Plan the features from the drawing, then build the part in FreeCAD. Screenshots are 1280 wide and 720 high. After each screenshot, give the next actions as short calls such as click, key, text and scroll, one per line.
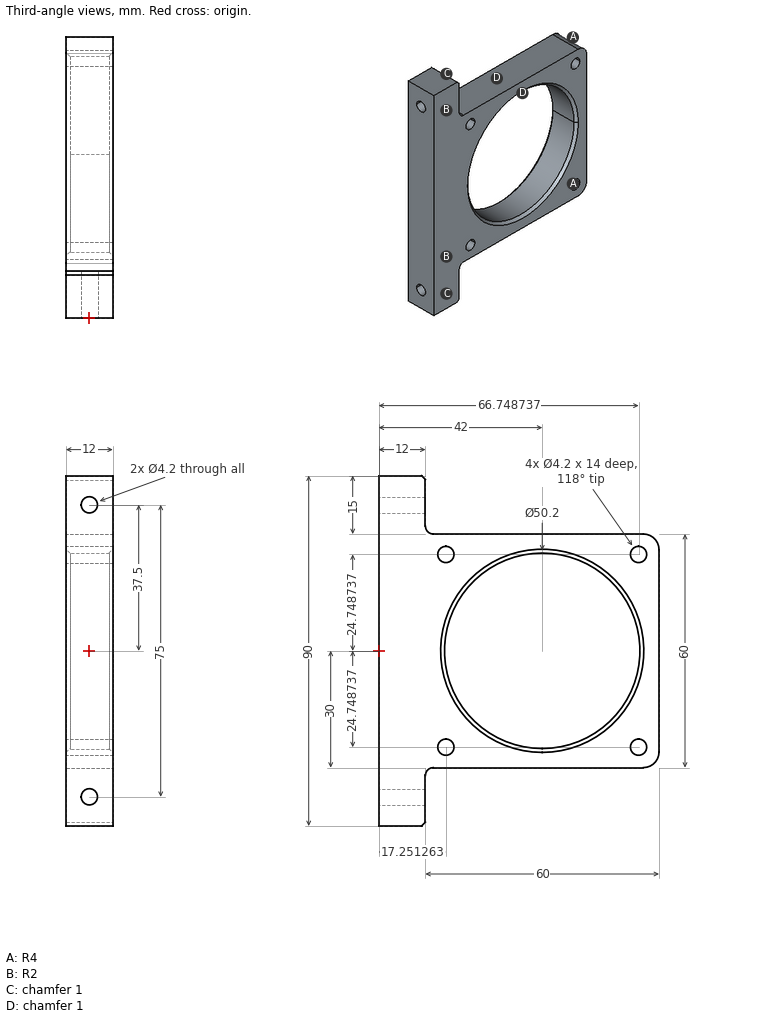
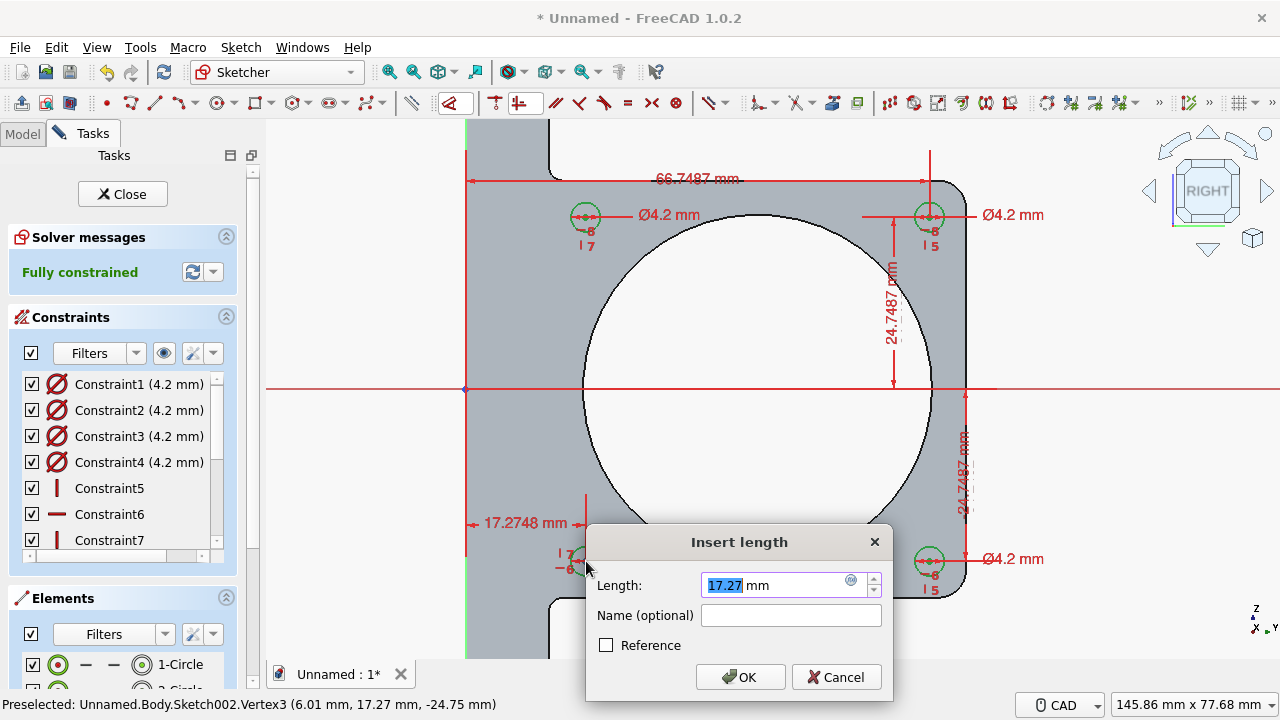
text(17.251263)
key(Return)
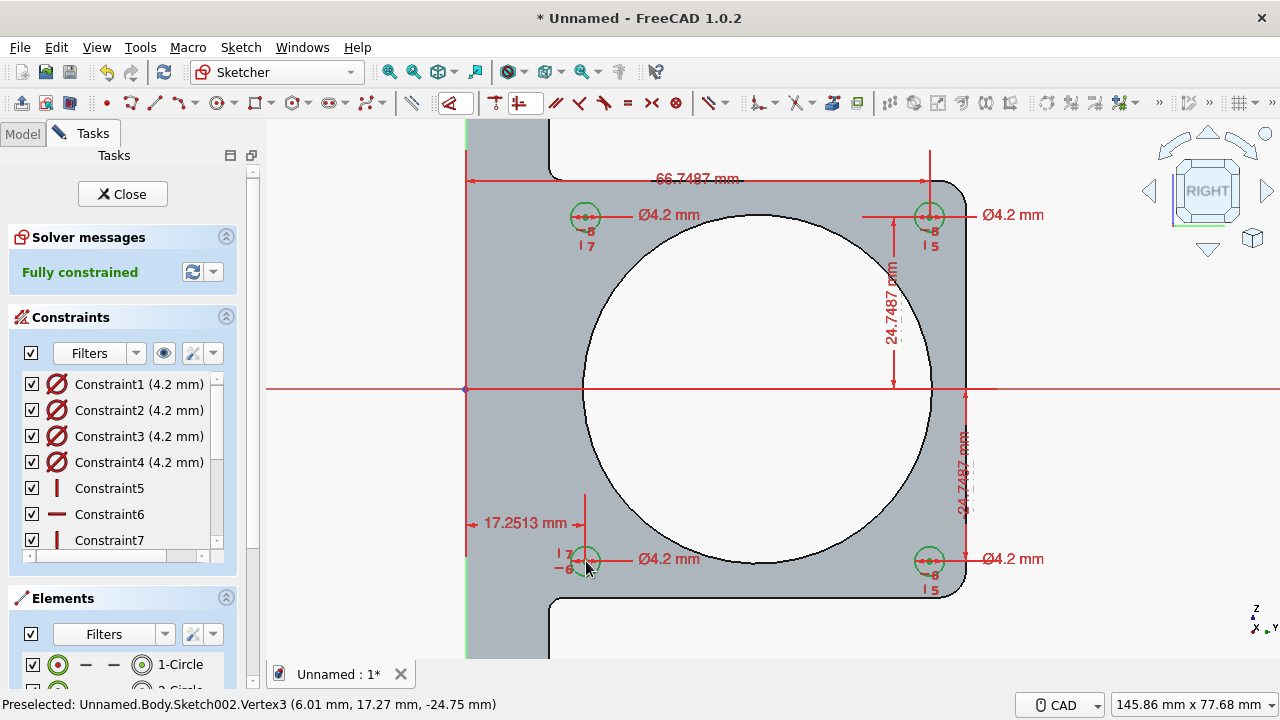
click(123, 194)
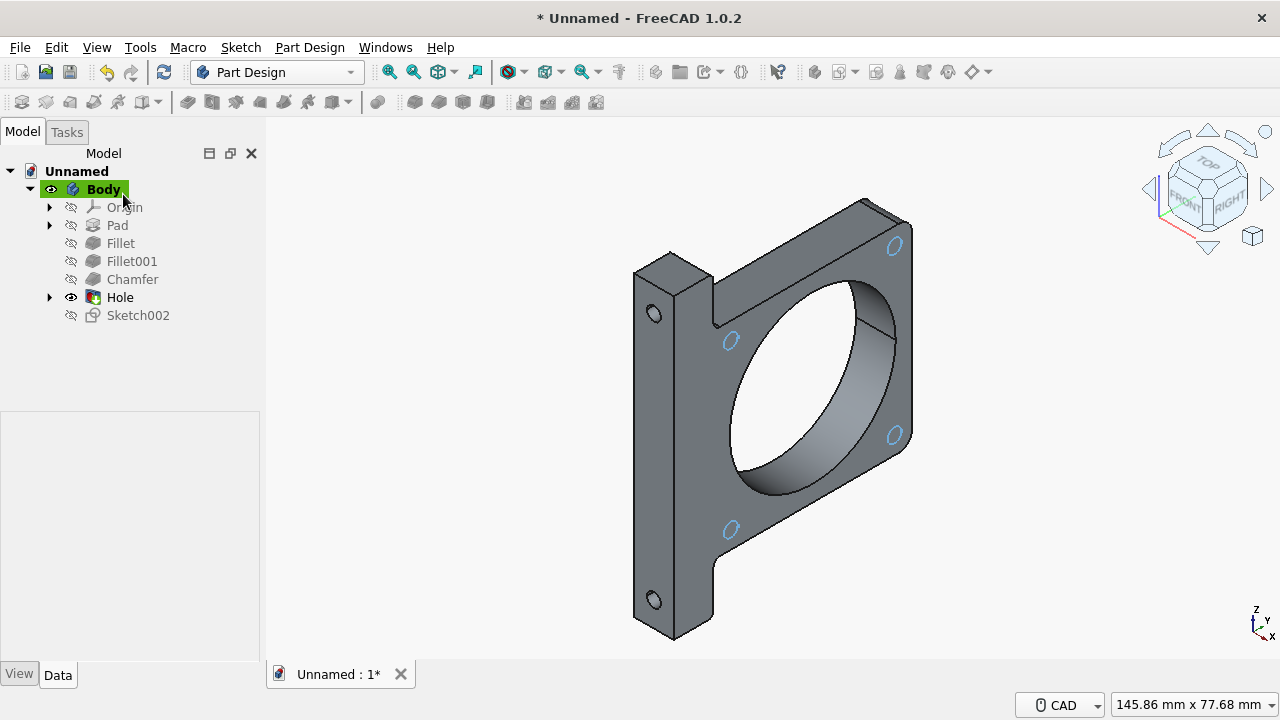
click(212, 102)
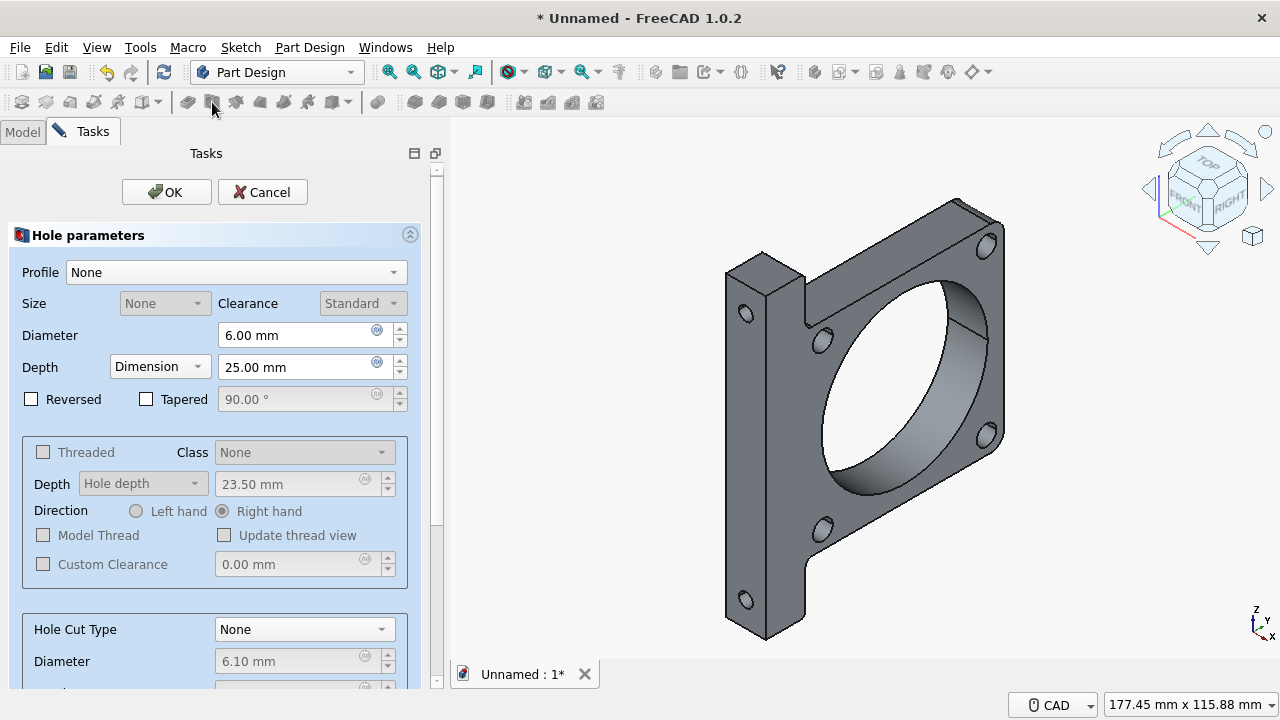
triple_click(305, 335)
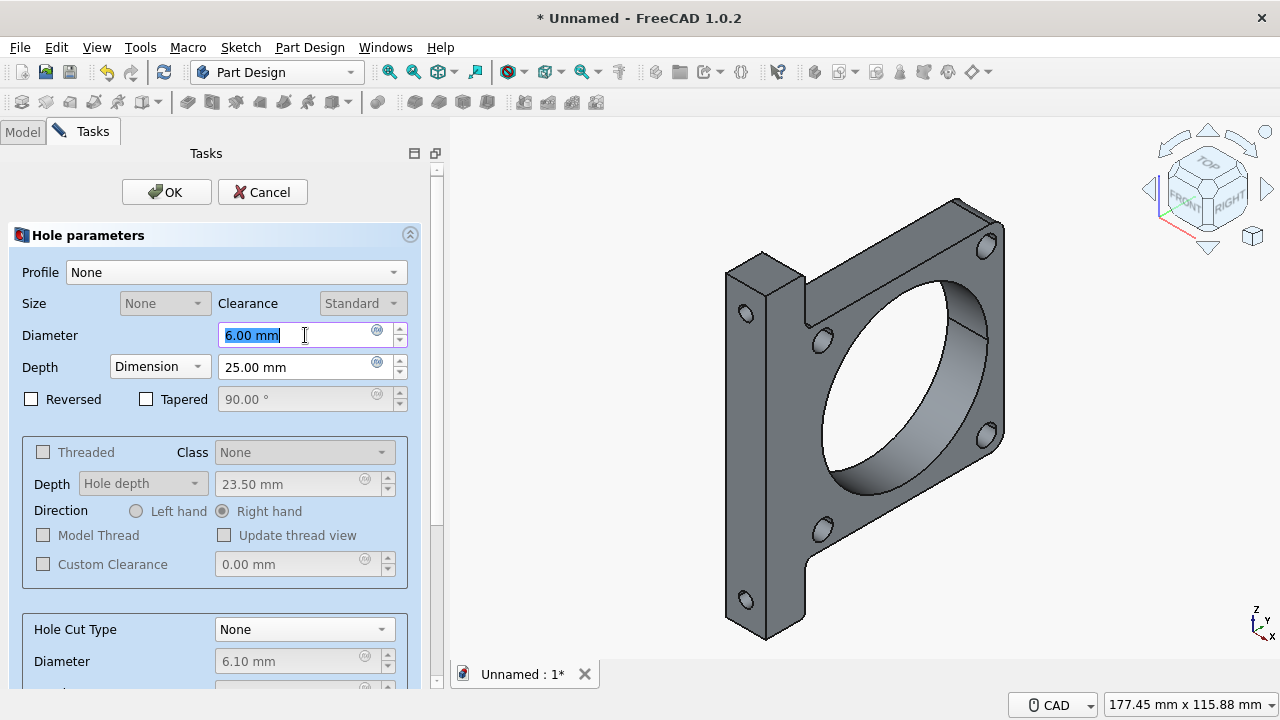
text(4.2)
key(Tab)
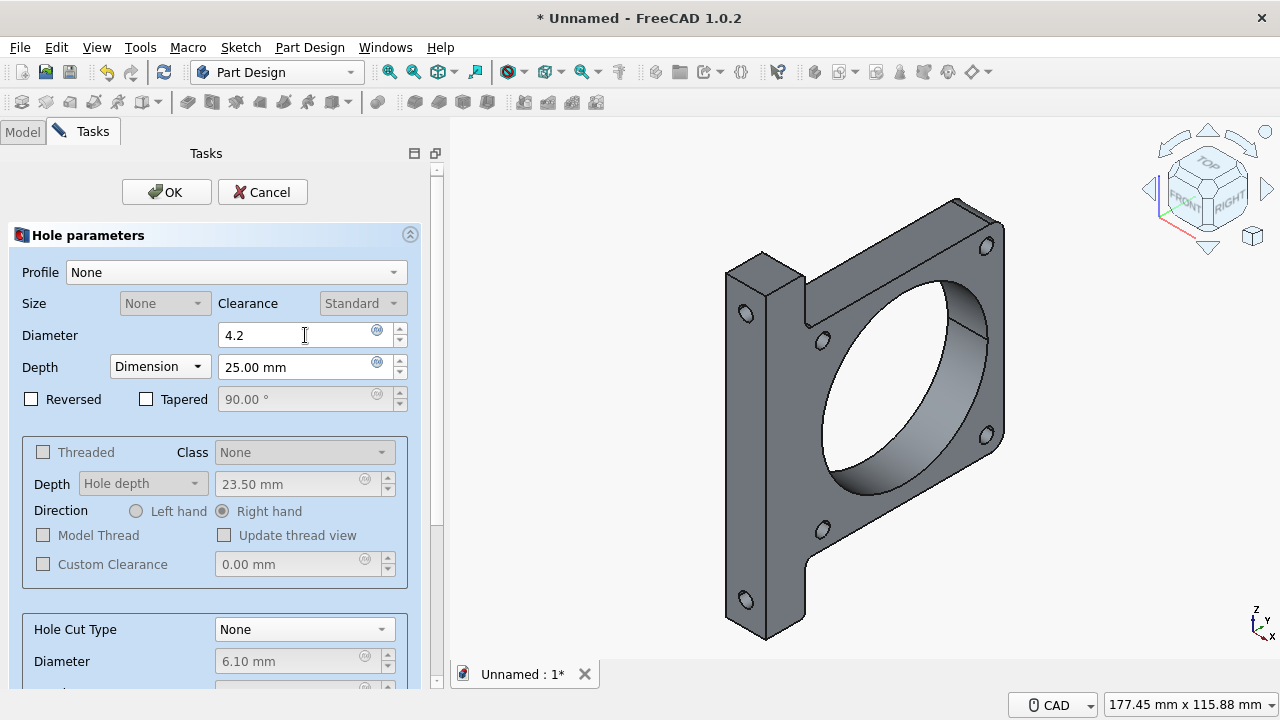
triple_click(305, 367)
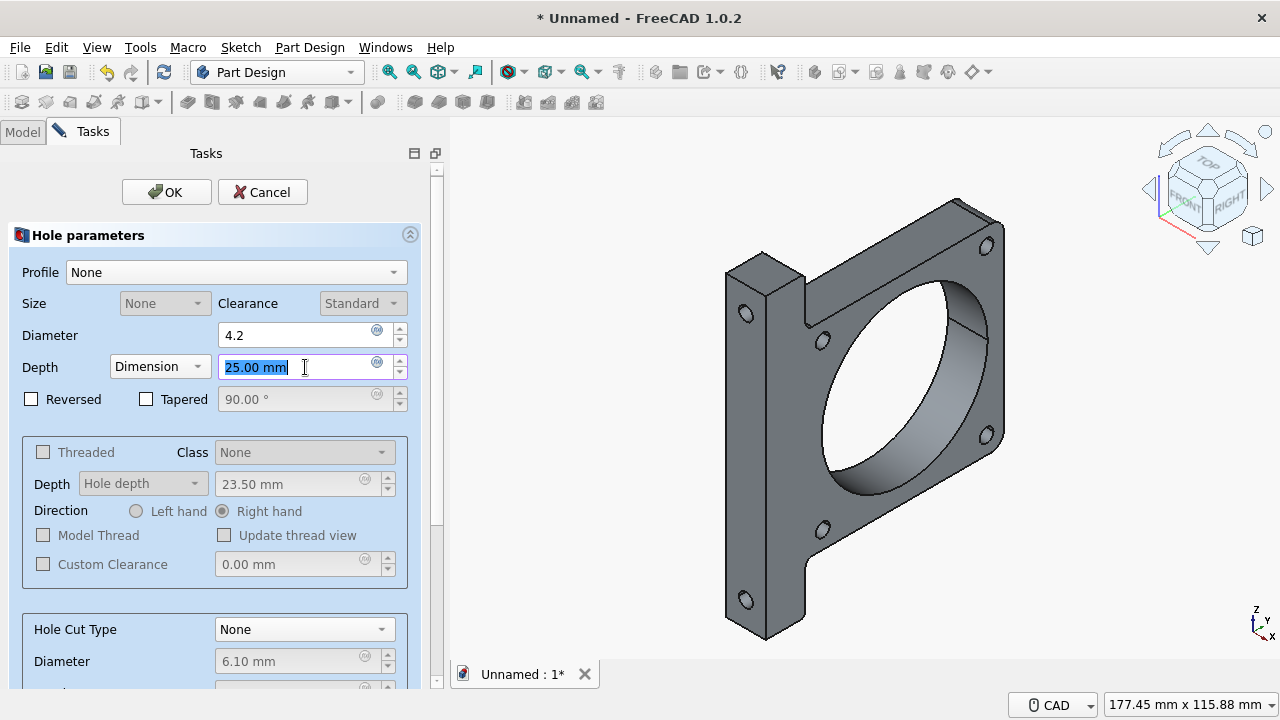
text(14)
key(Tab)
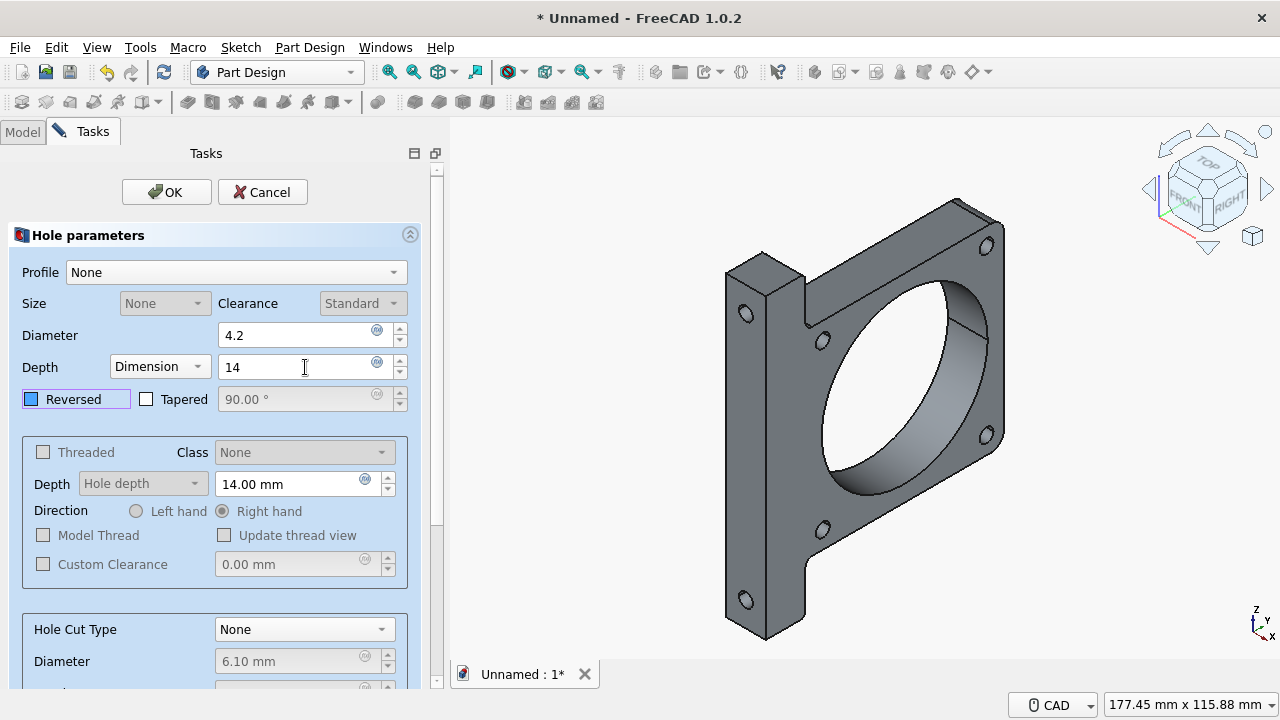
click(167, 192)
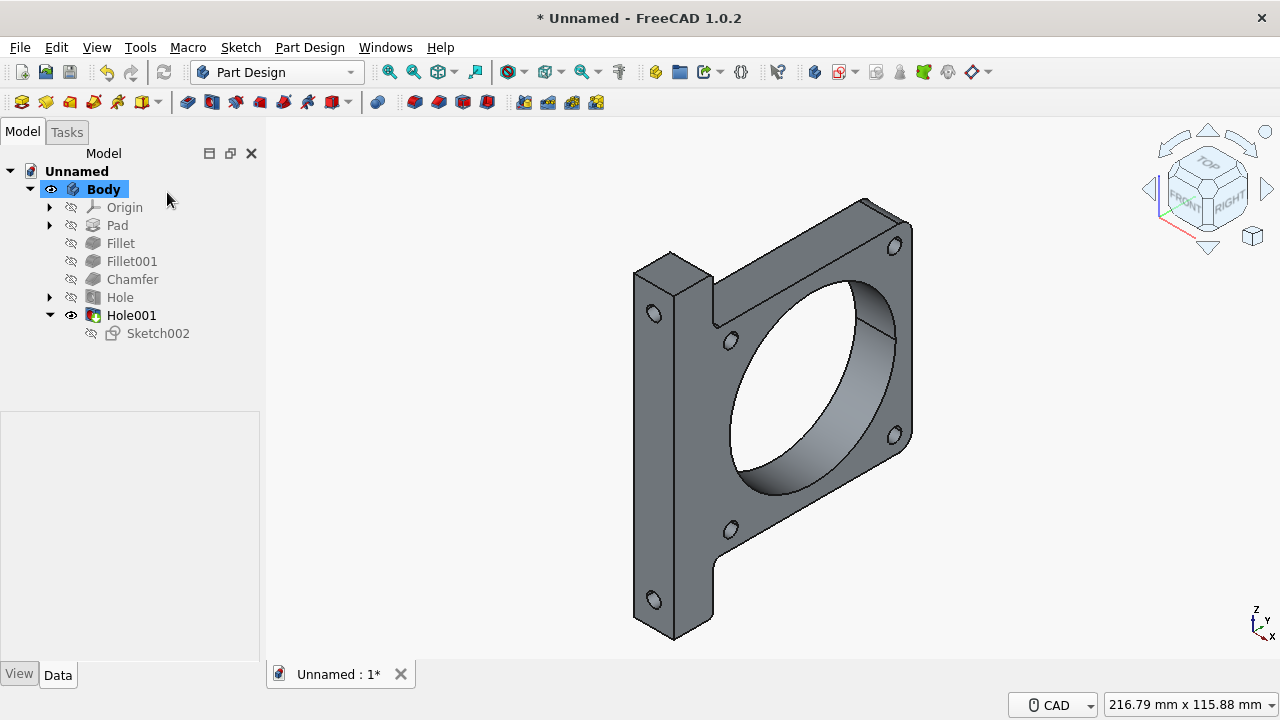
click(746, 482)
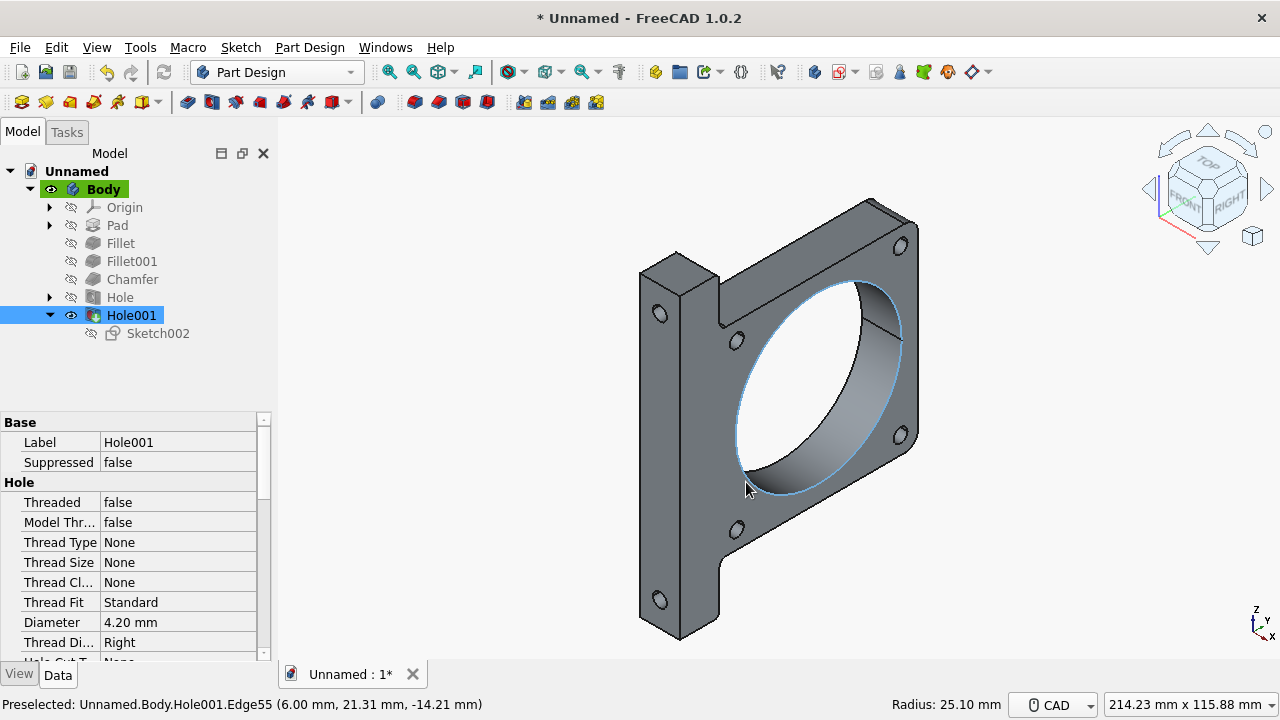
key(2)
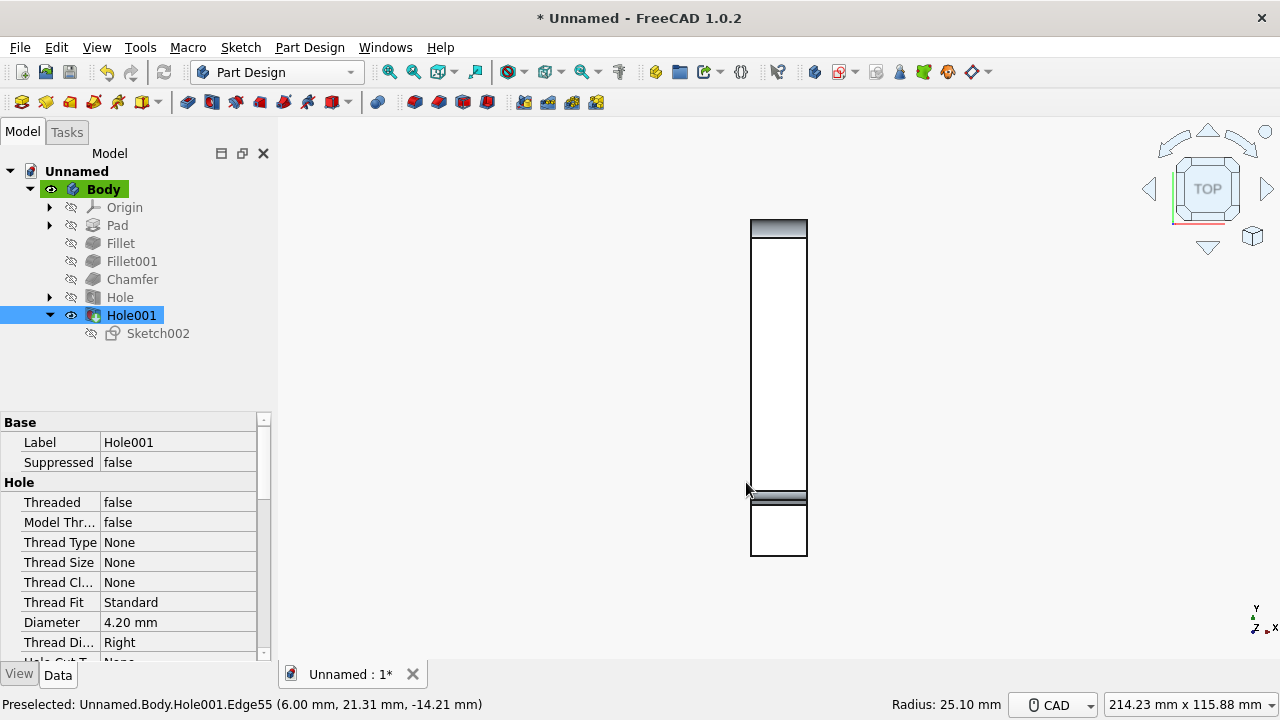
key(0)